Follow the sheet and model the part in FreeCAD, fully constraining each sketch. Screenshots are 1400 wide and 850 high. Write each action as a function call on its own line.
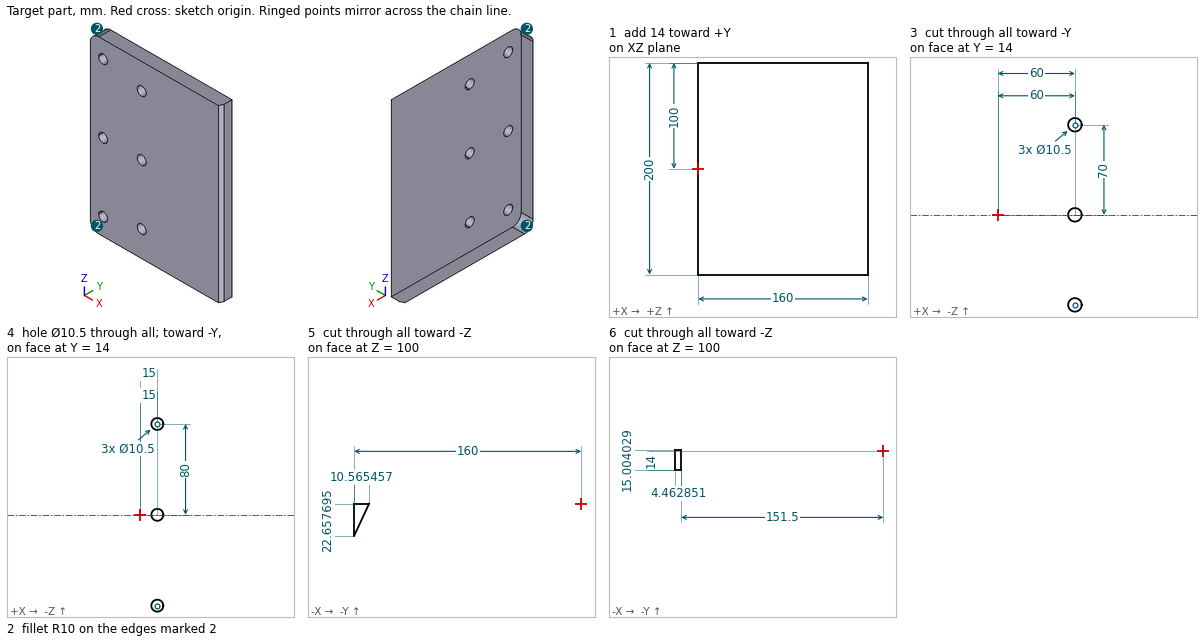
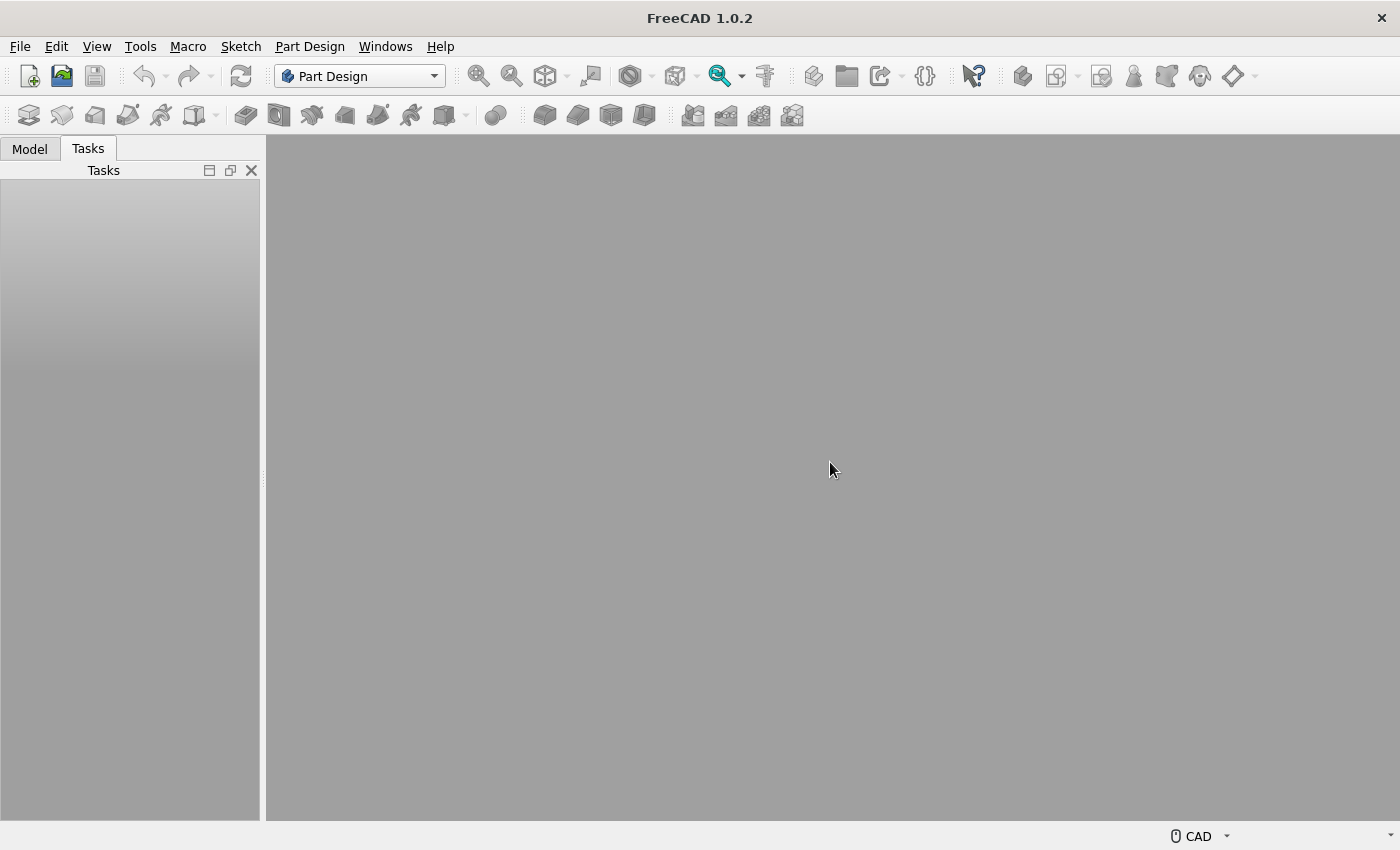
click(29, 76)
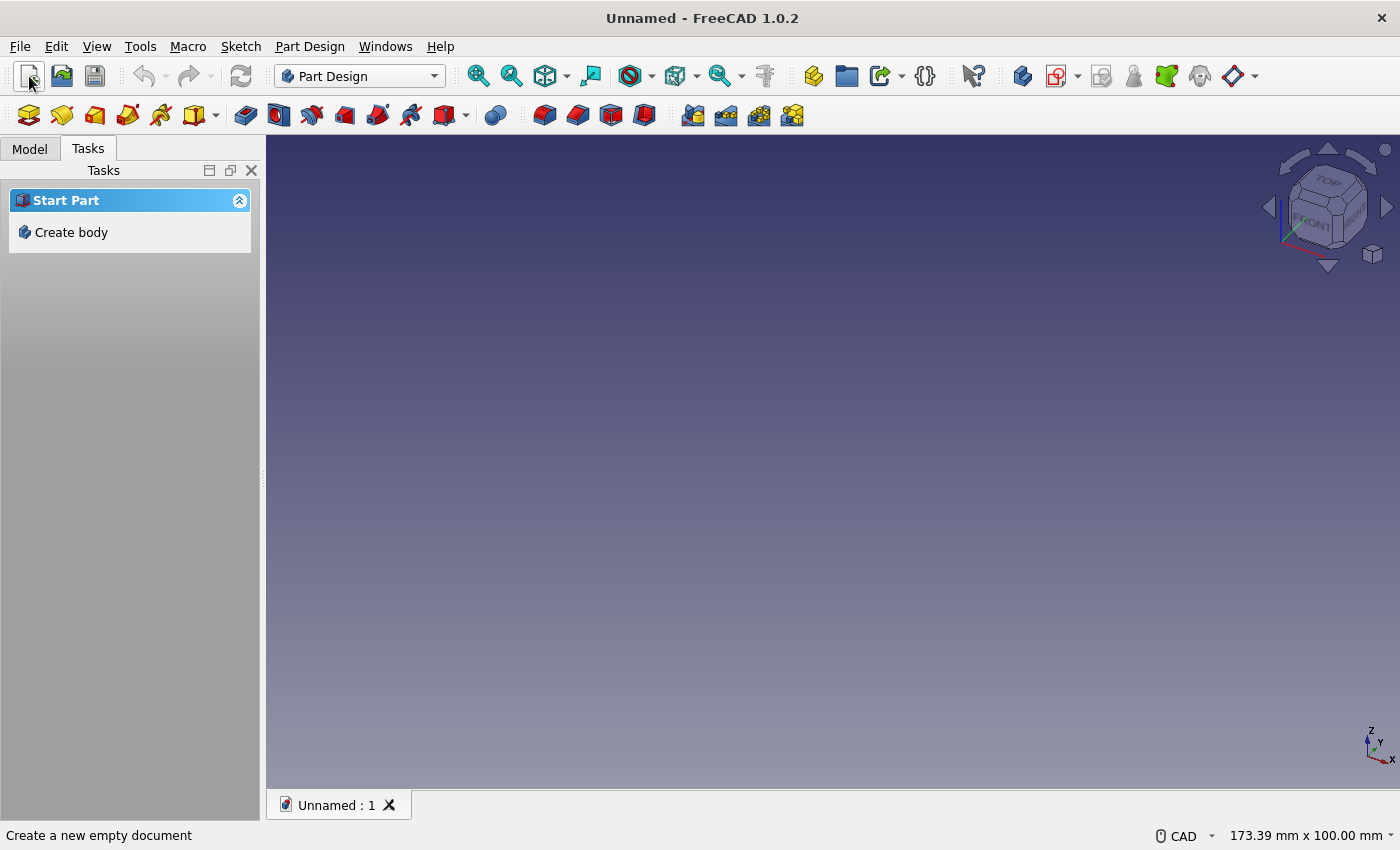
click(1056, 76)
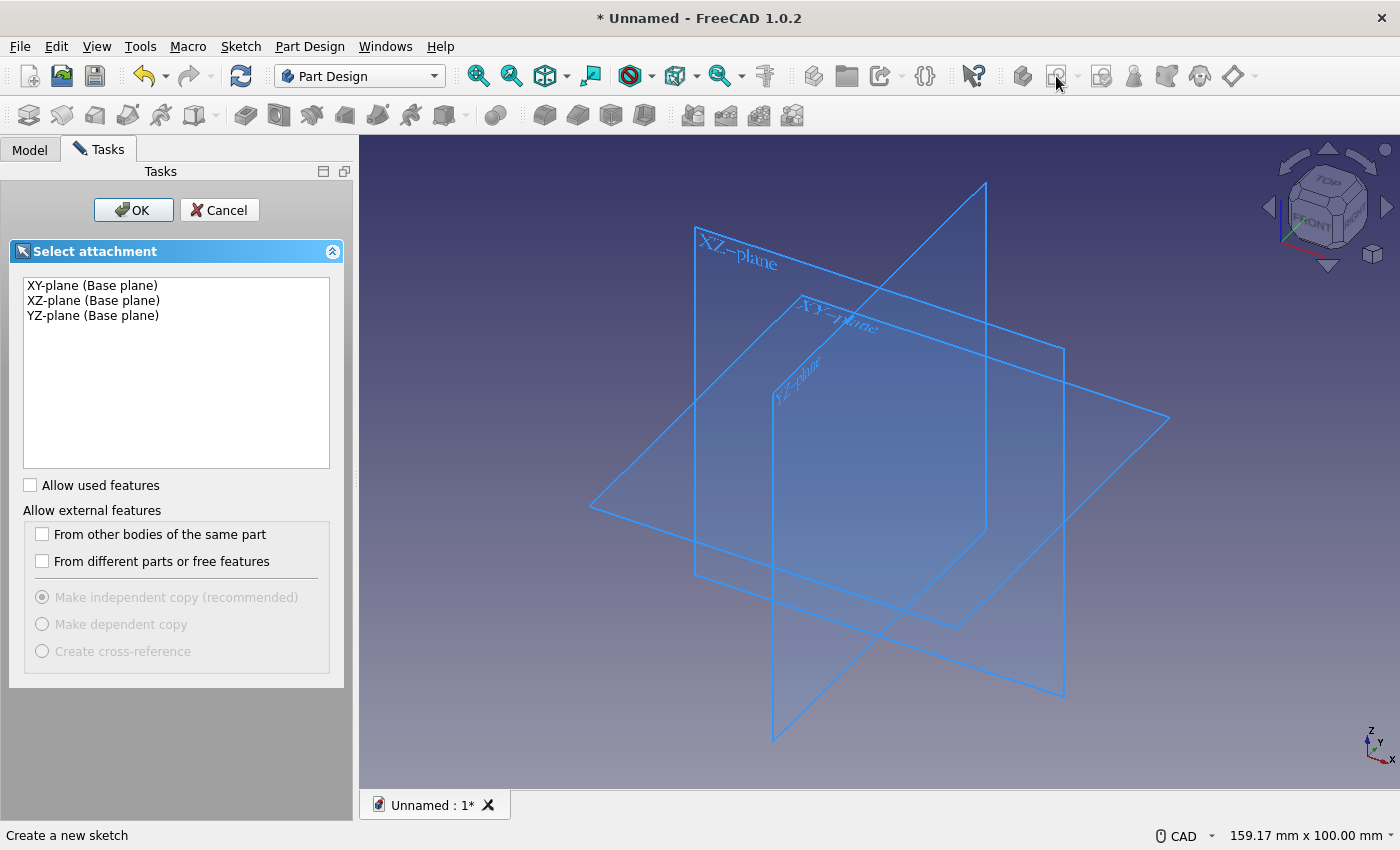
click(84, 300)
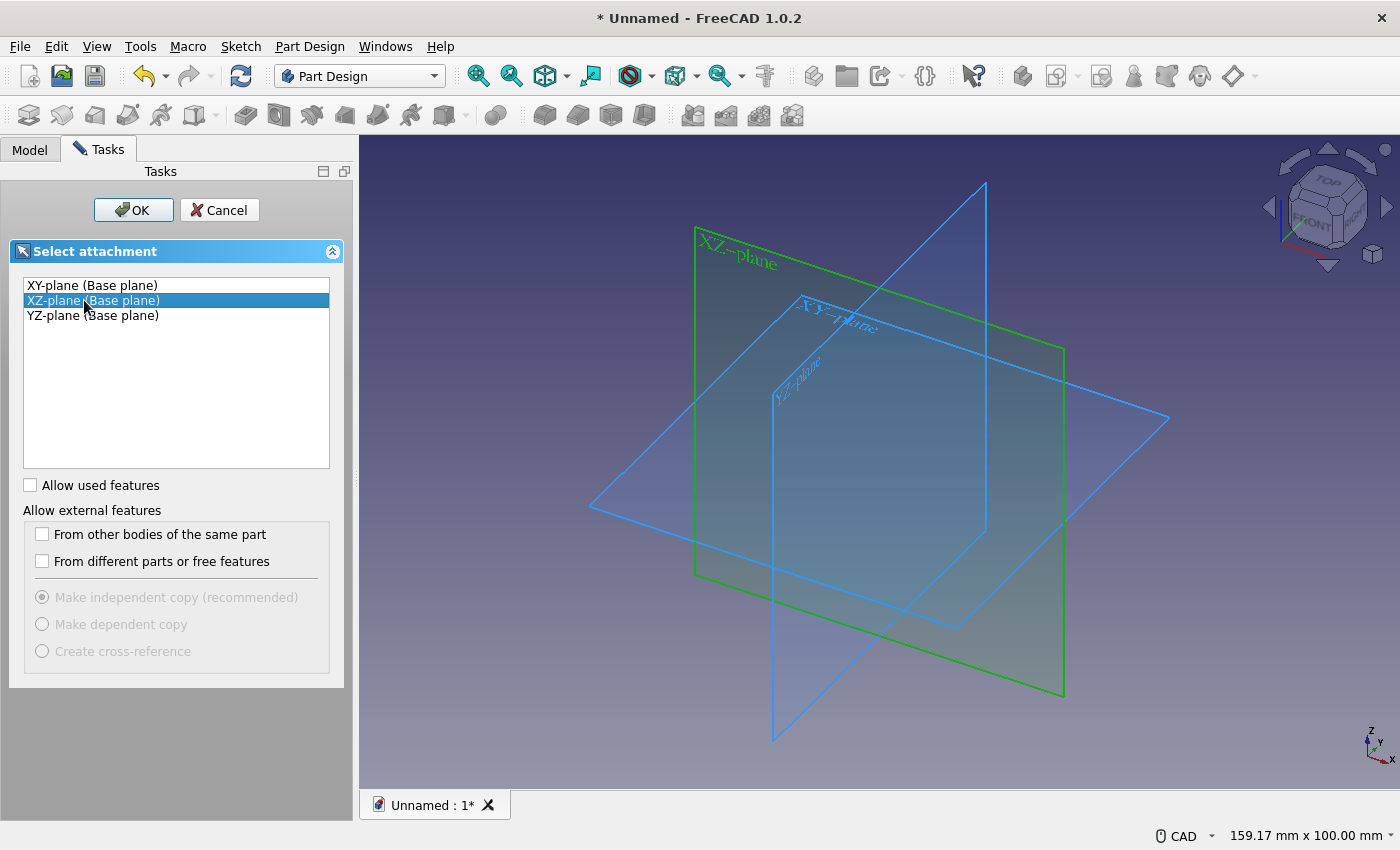
click(134, 210)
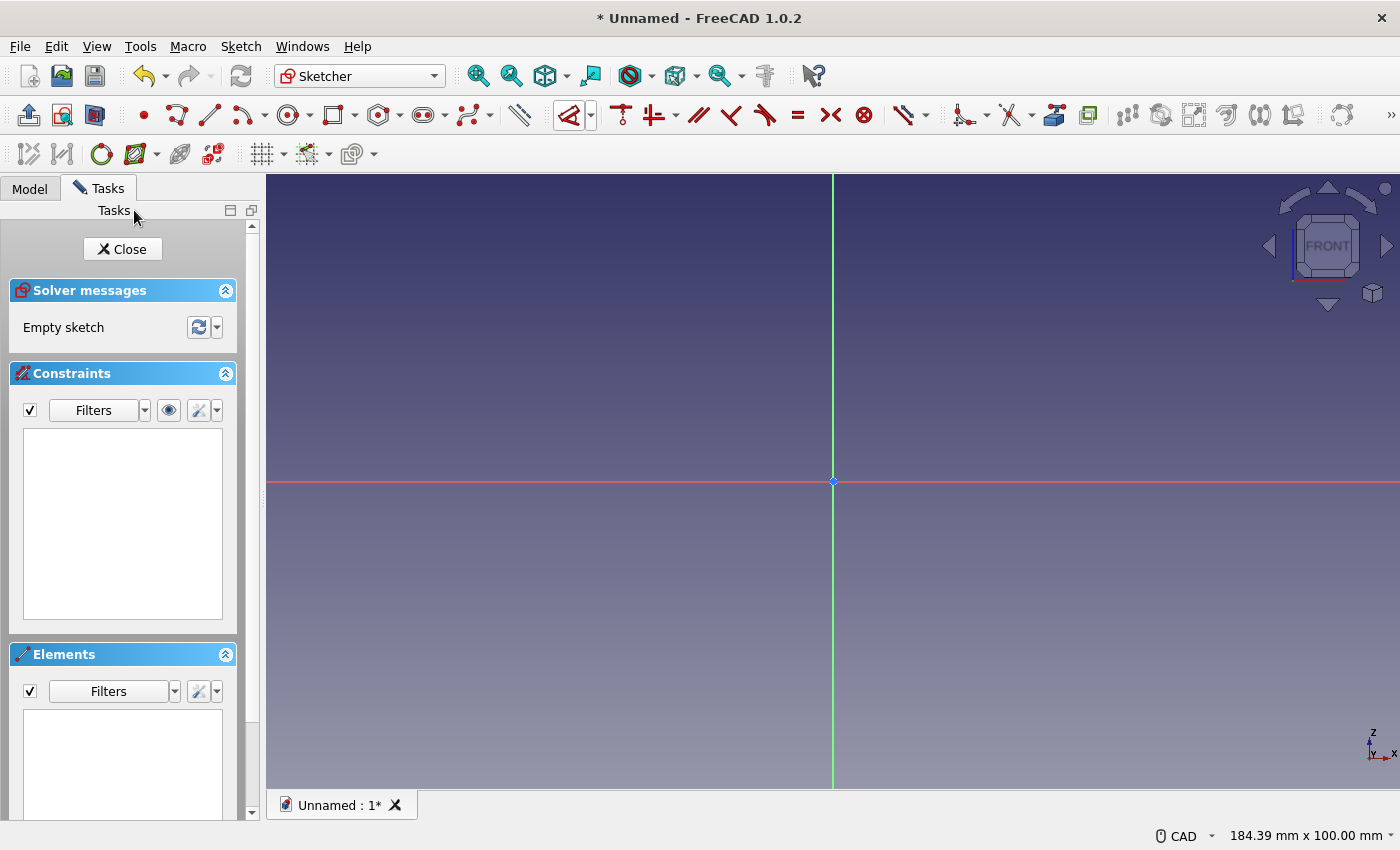
scroll(523, 481, down, 6)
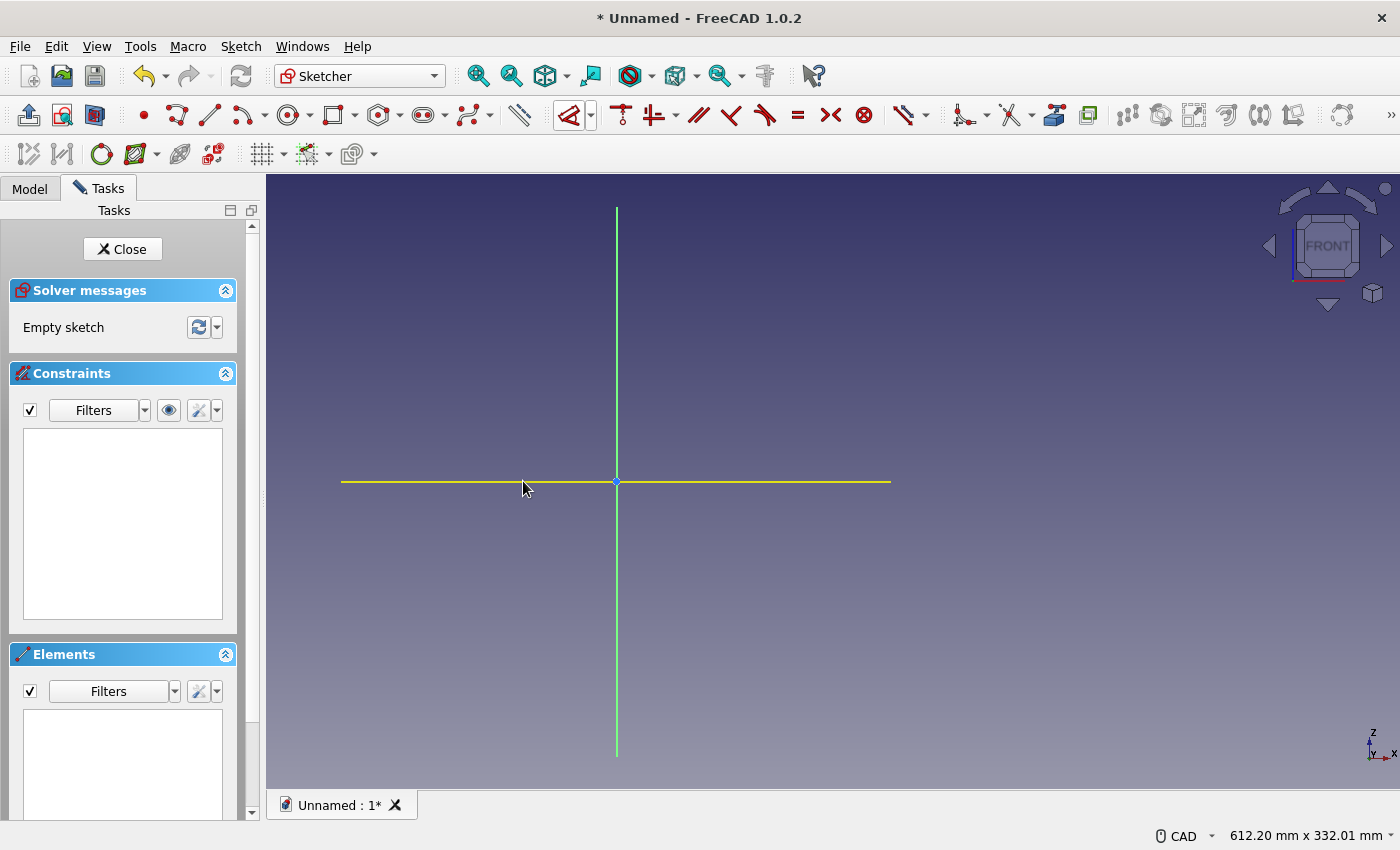
key(g)
key(r)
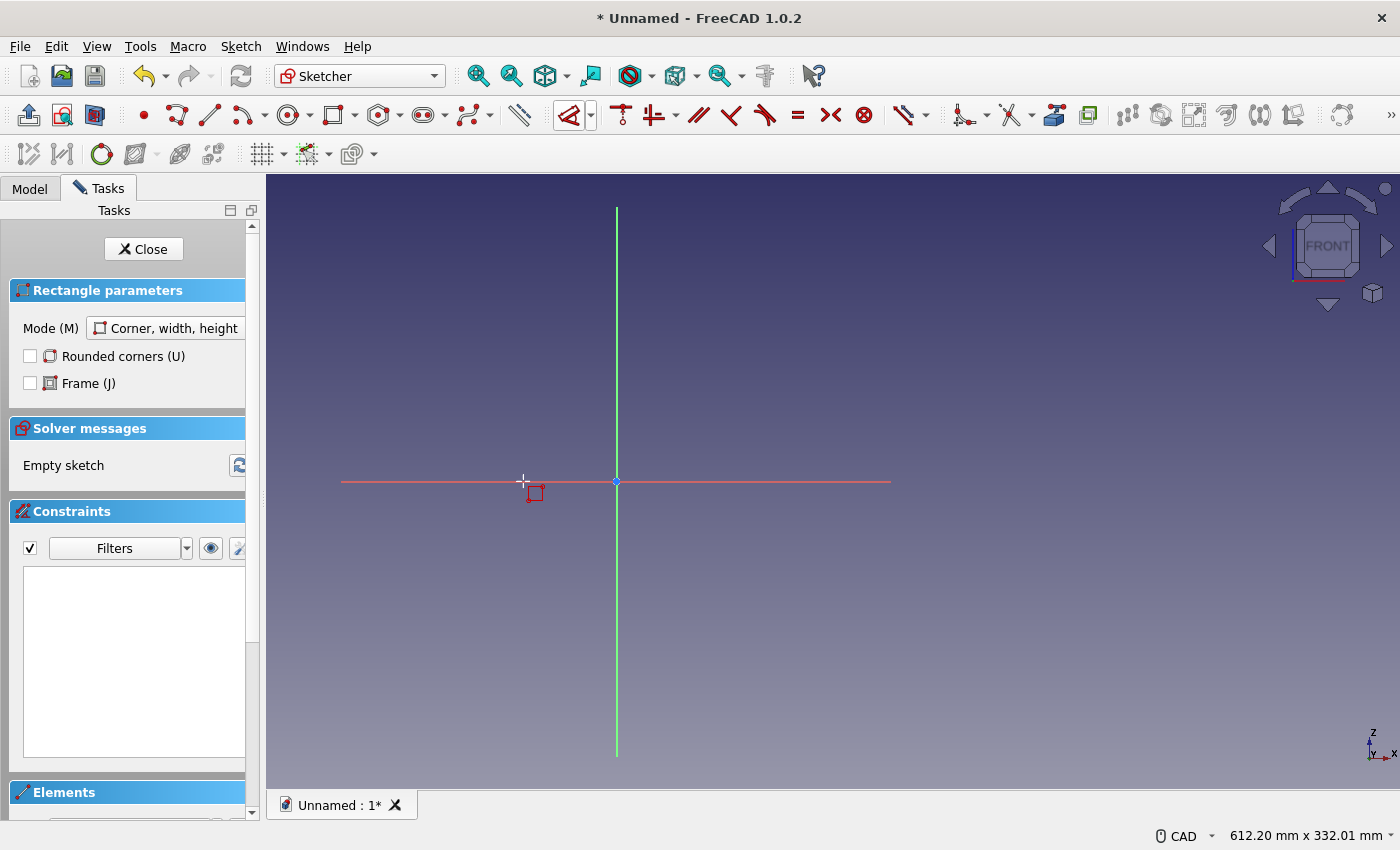
click(617, 296)
click(913, 667)
key(Escape)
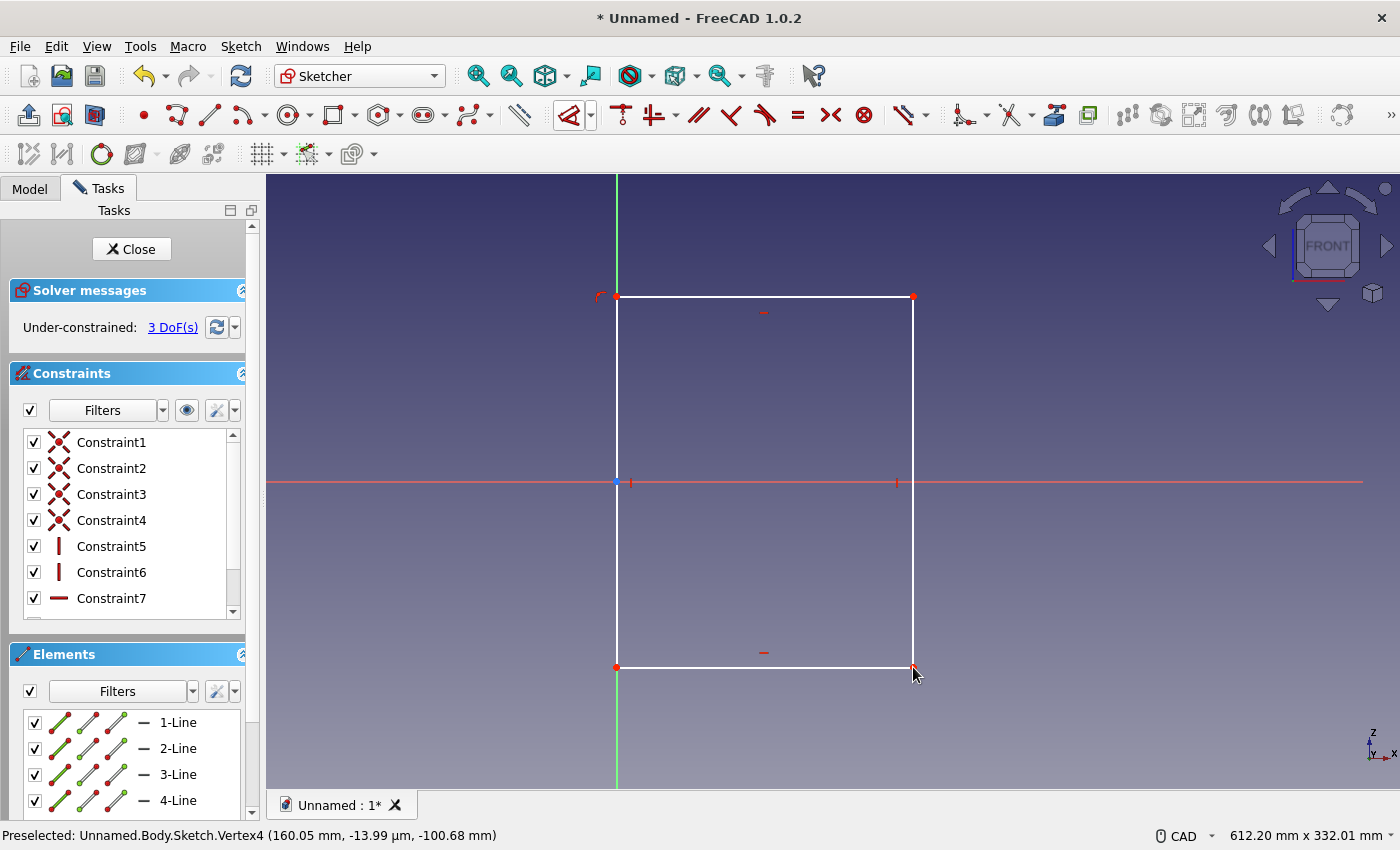
key(d)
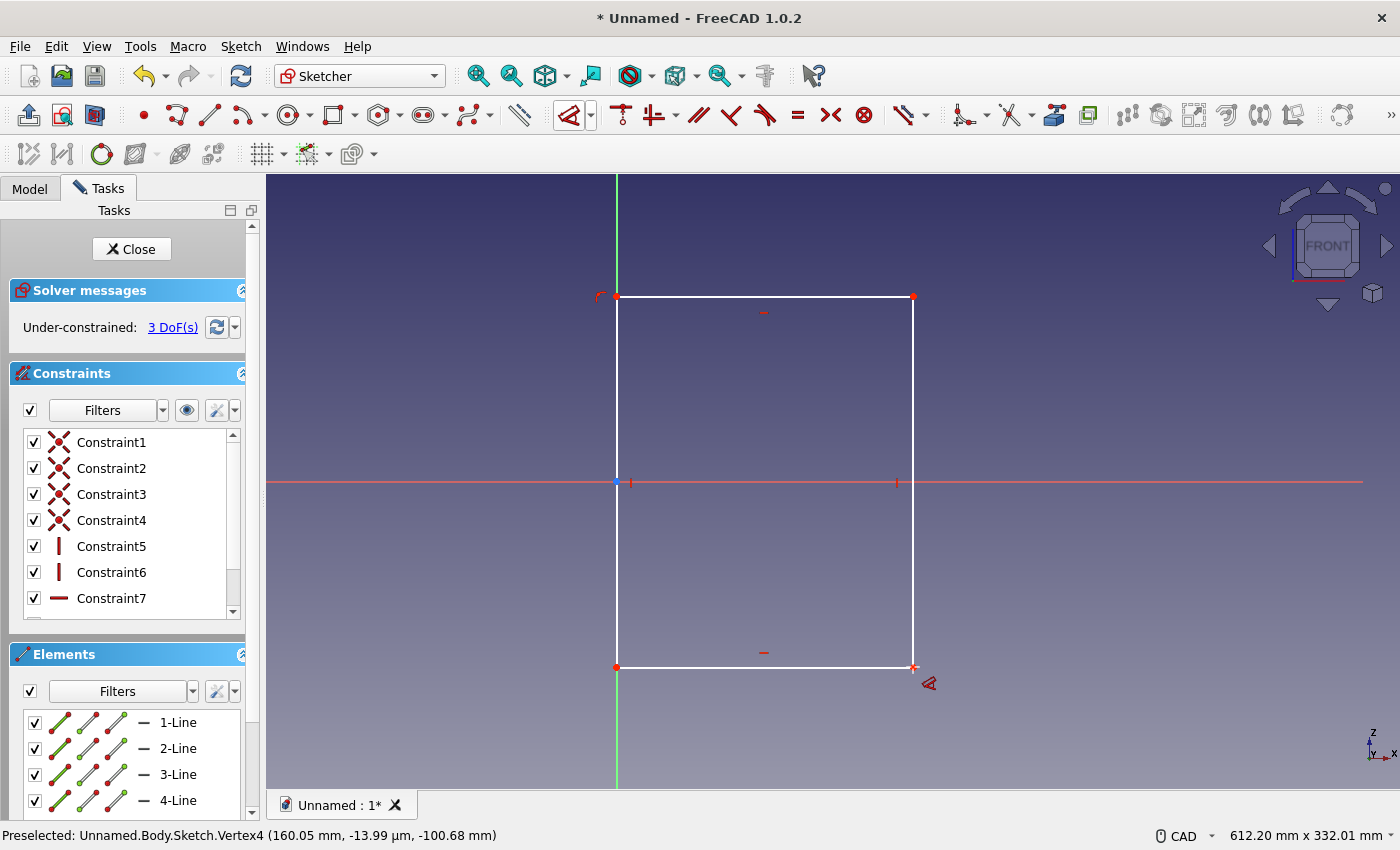
click(617, 408)
click(583, 397)